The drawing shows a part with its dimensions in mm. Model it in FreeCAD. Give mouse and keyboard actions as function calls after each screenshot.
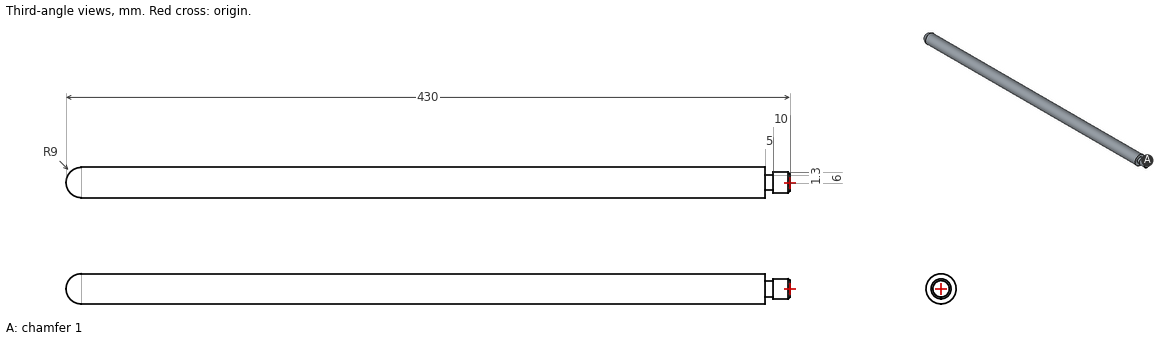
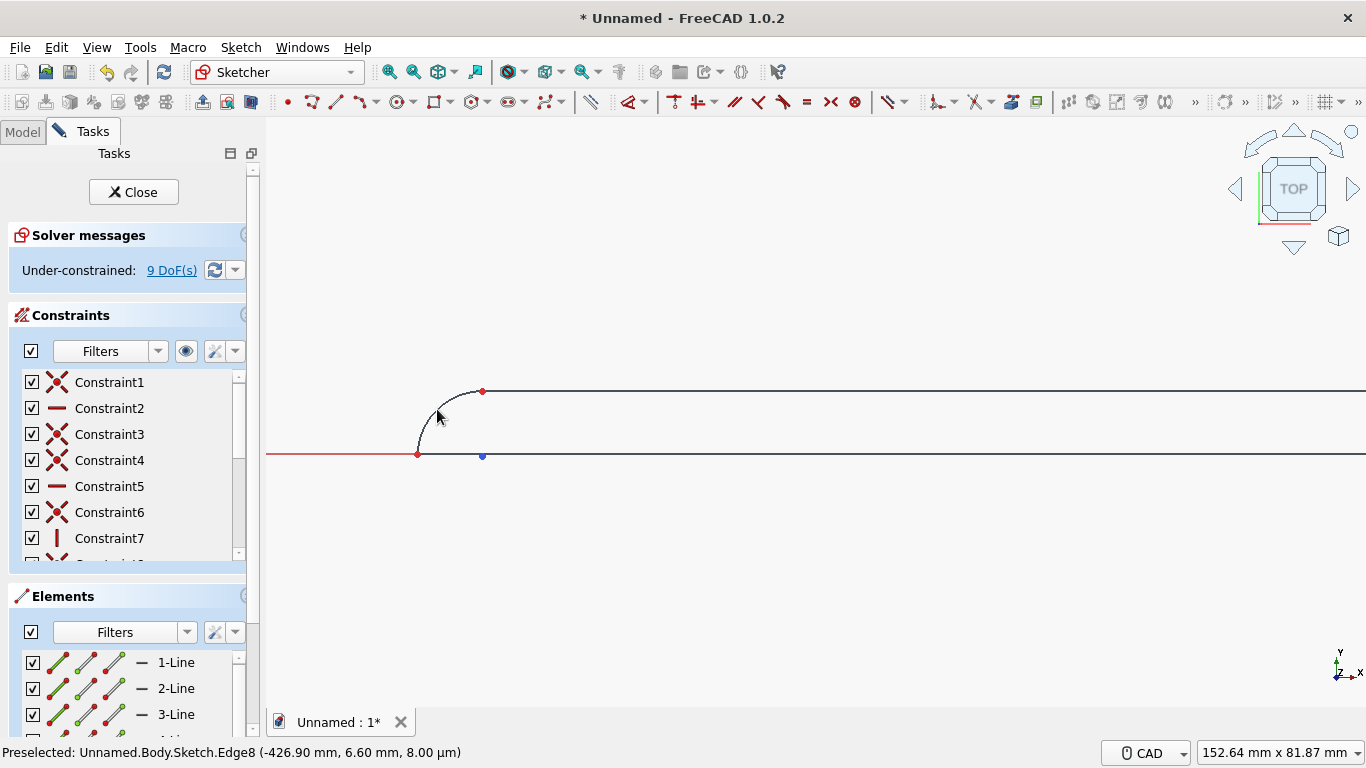
scroll(439, 409, down, 8)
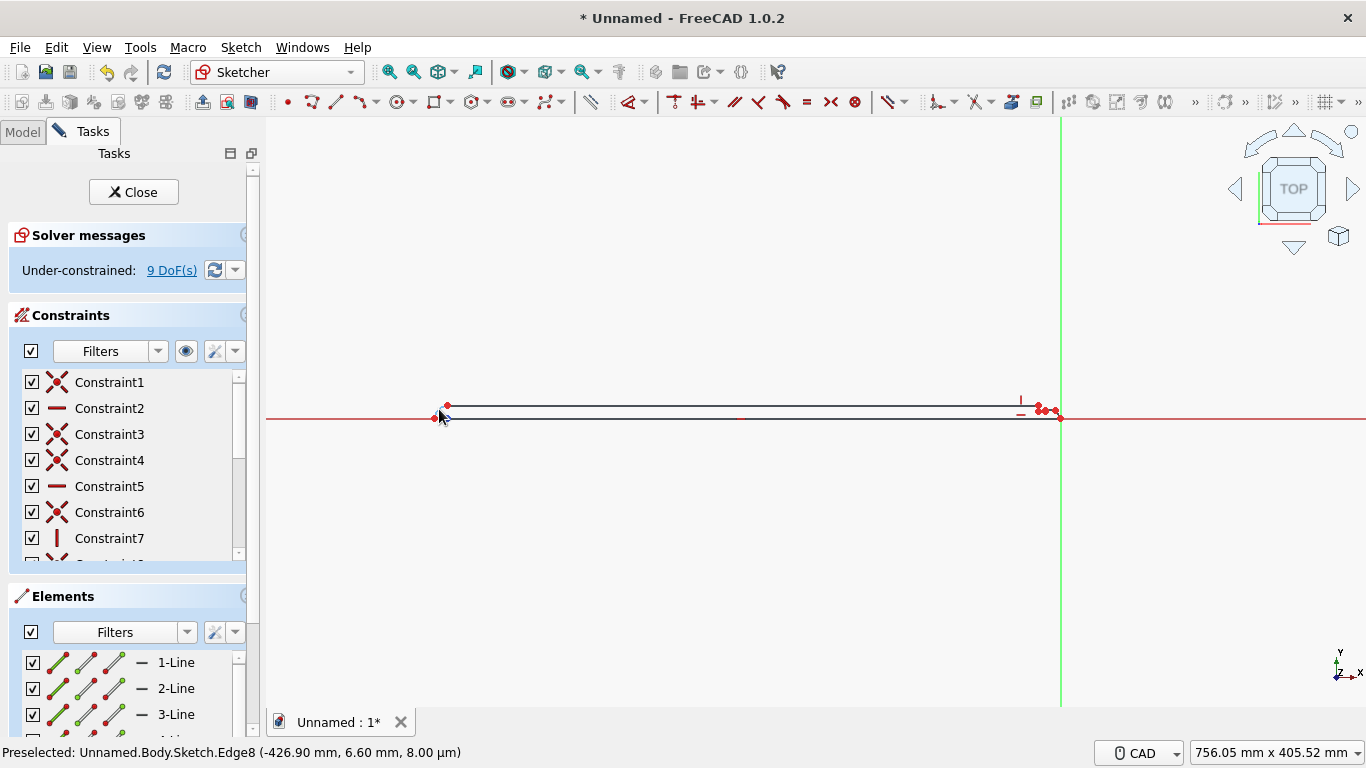
click(566, 406)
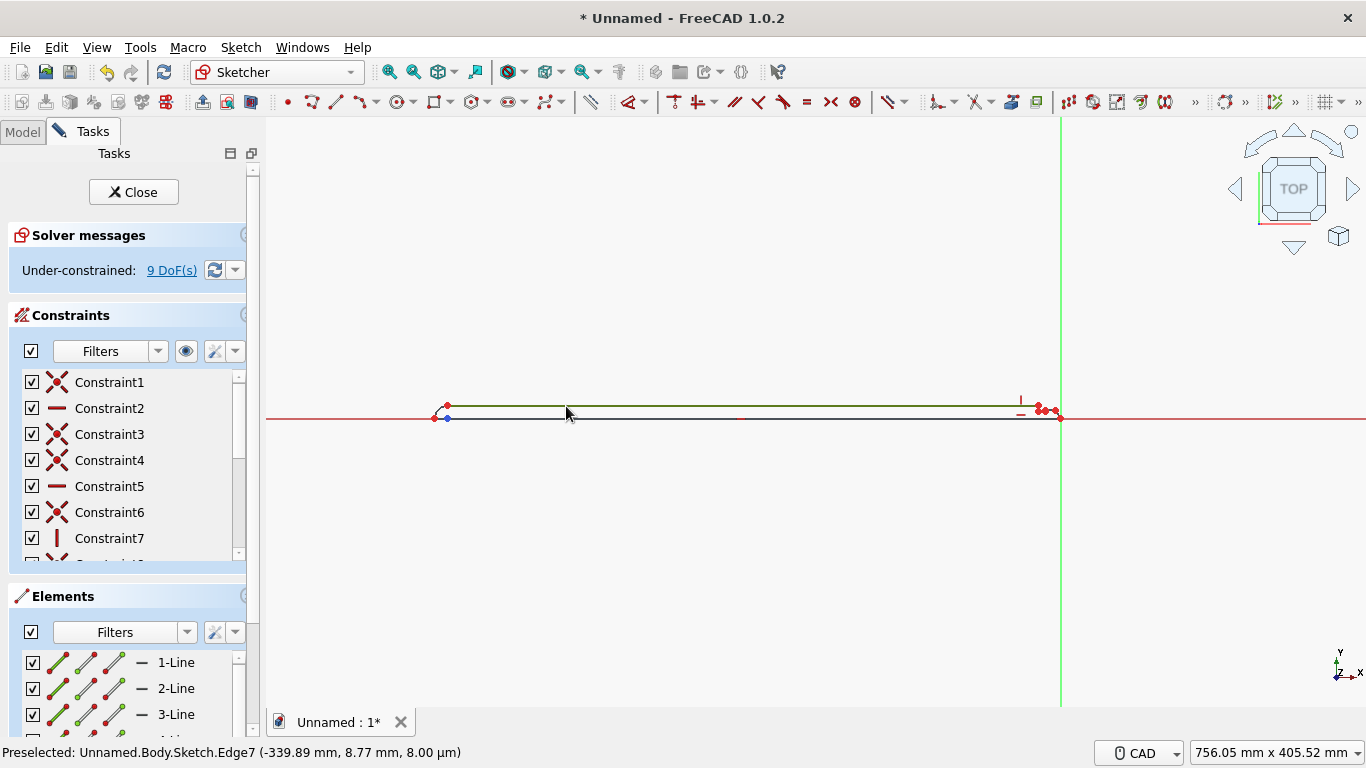
scroll(439, 410, up, 3)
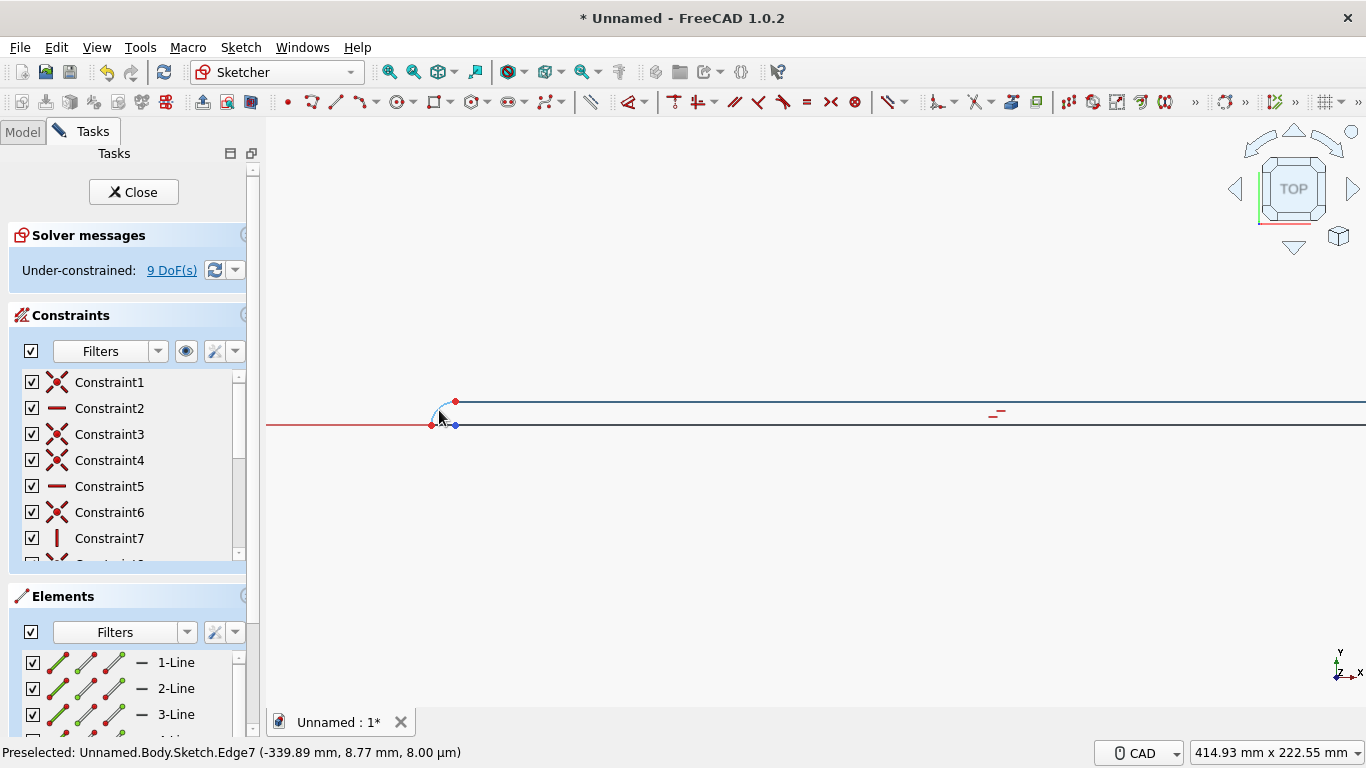
click(439, 409)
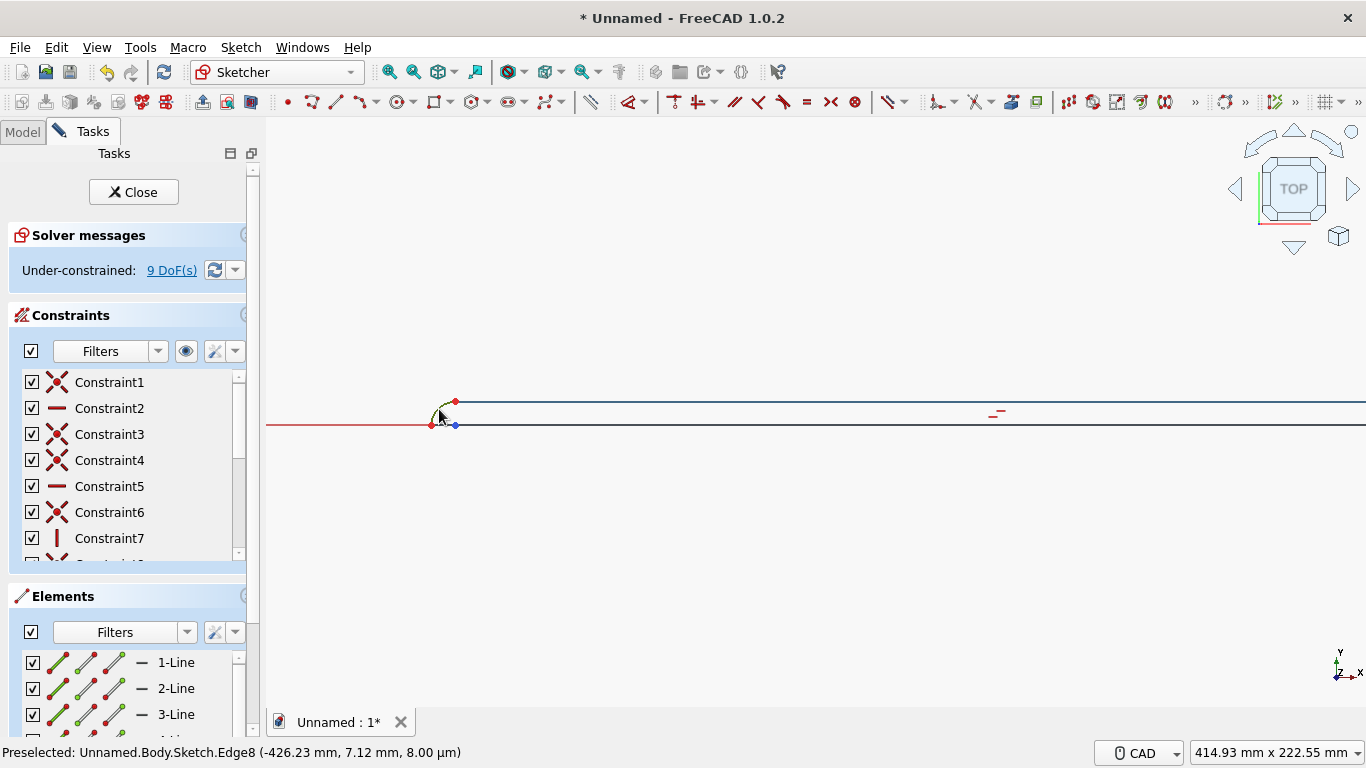
click(784, 102)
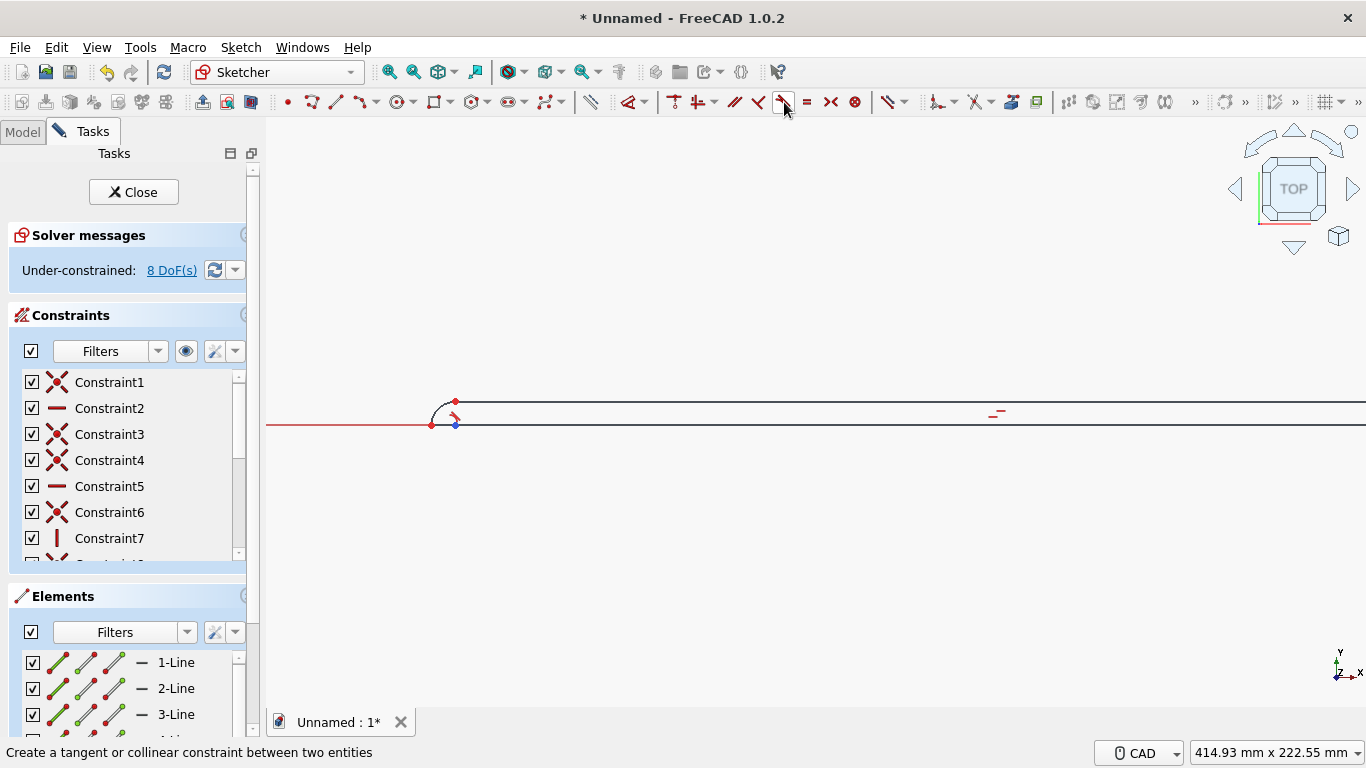
scroll(439, 410, down, 3)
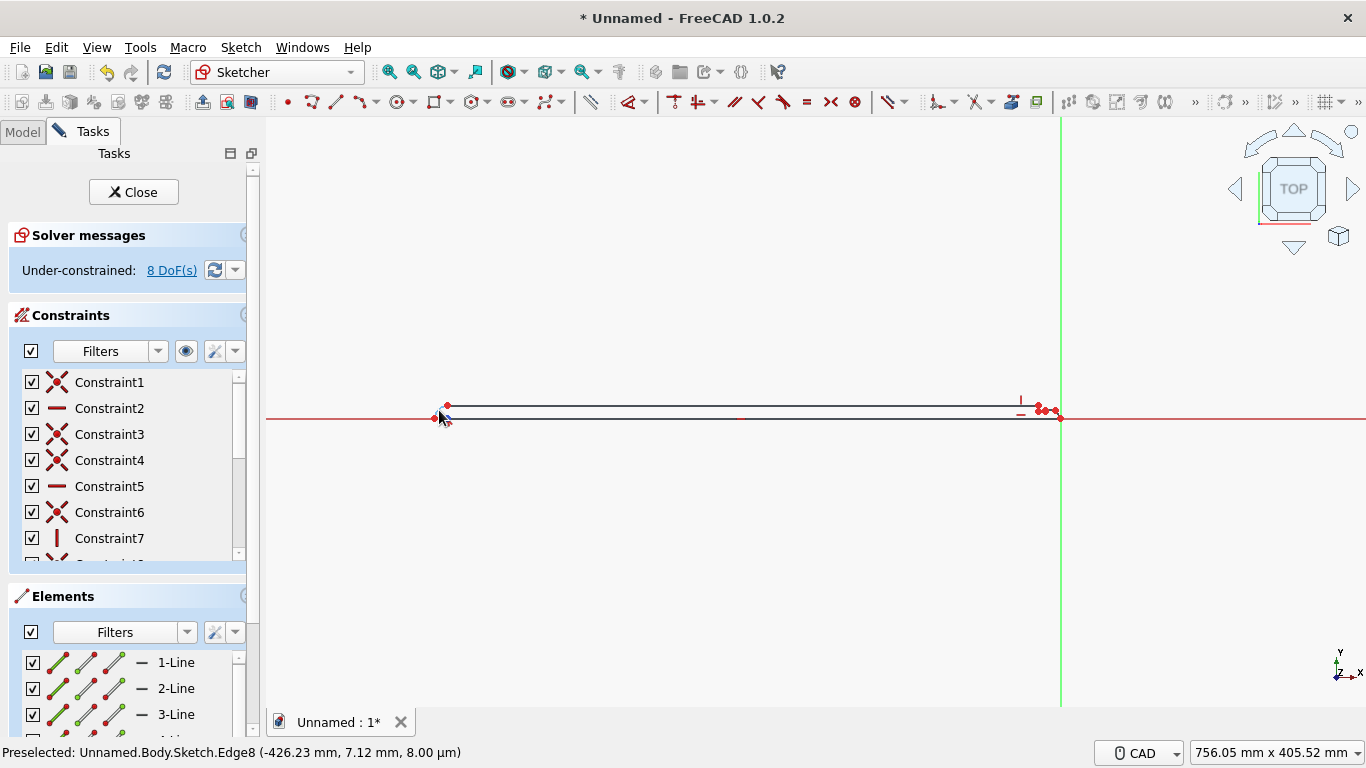
scroll(1059, 415, up, 8)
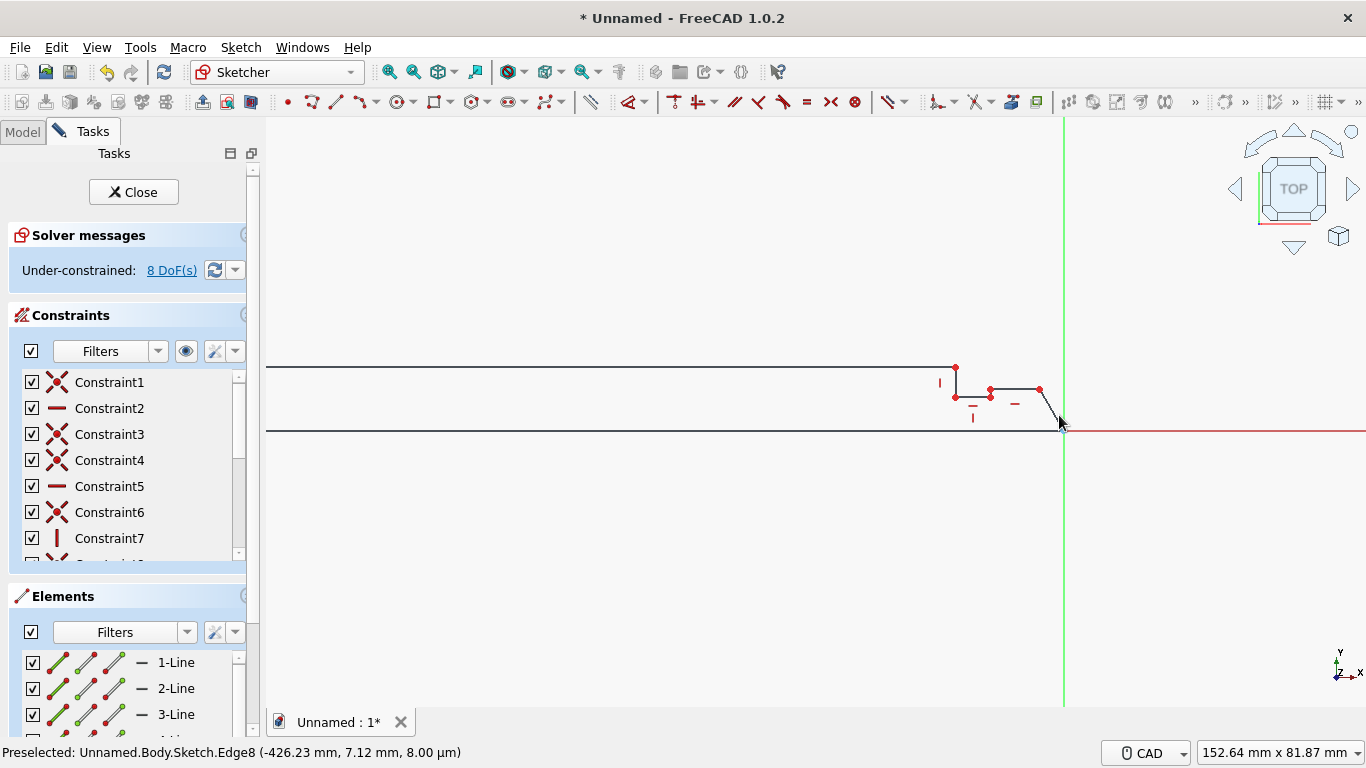
click(1054, 414)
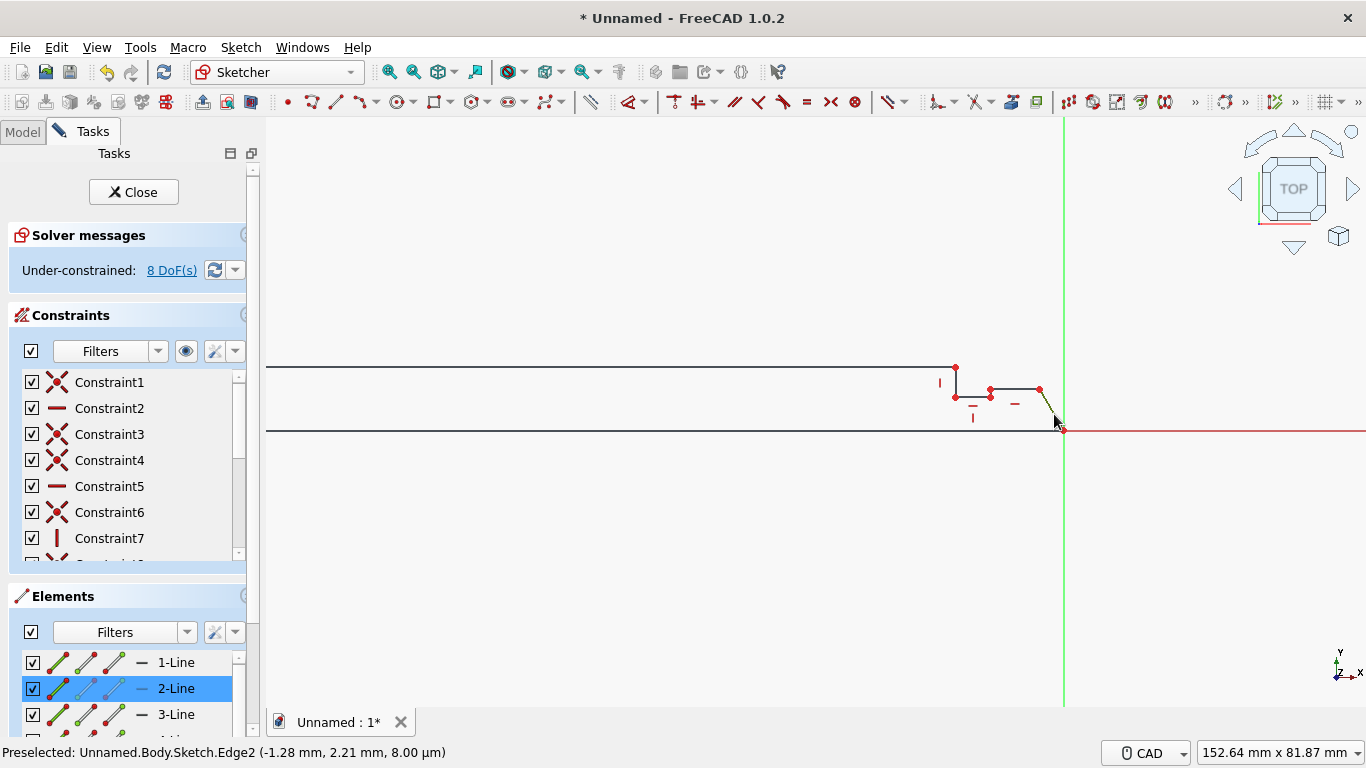
click(716, 102)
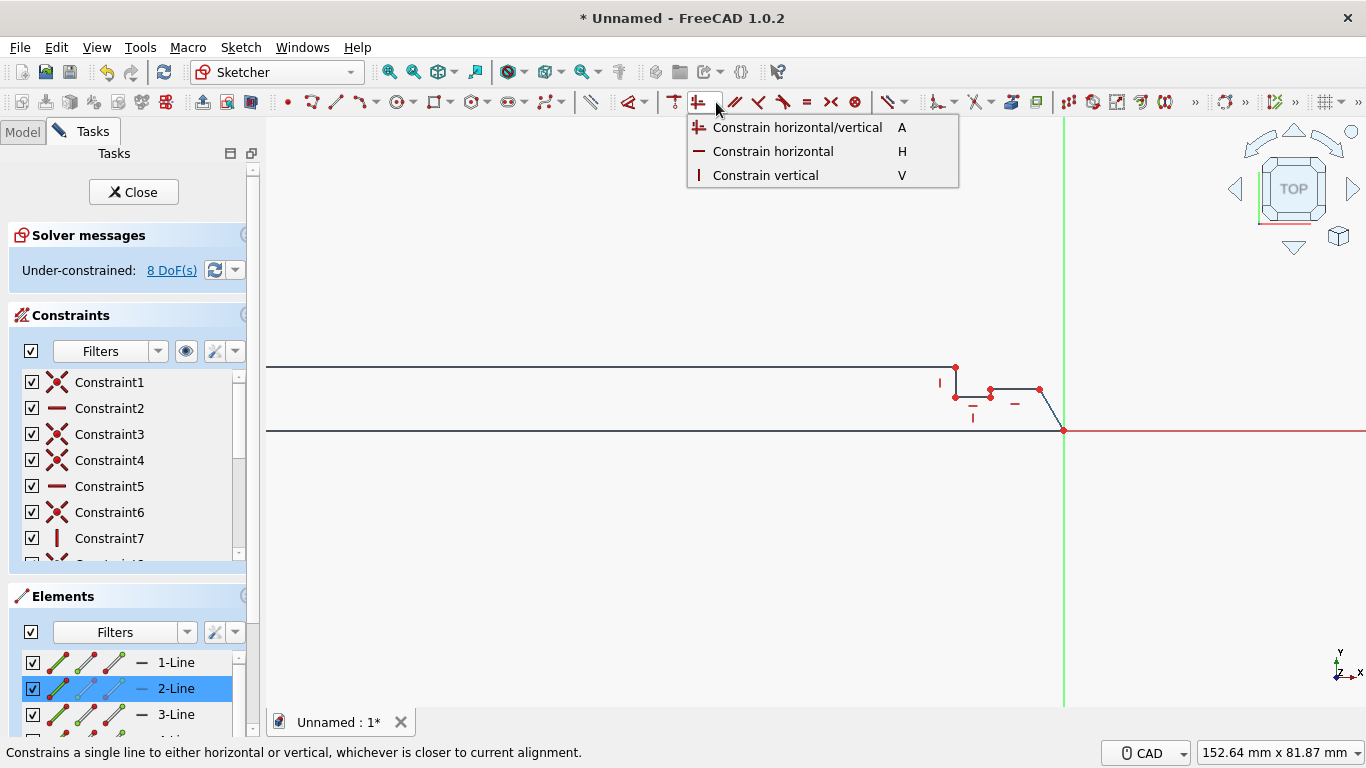
click(823, 175)